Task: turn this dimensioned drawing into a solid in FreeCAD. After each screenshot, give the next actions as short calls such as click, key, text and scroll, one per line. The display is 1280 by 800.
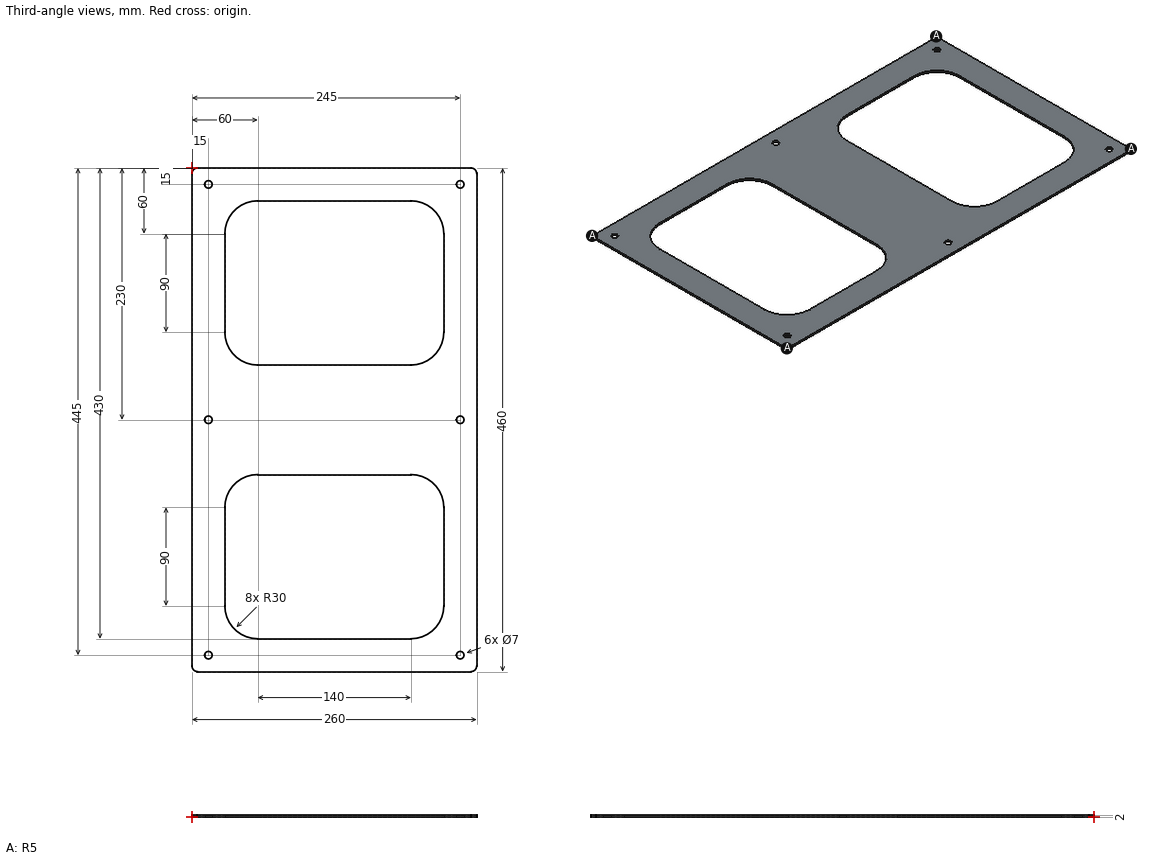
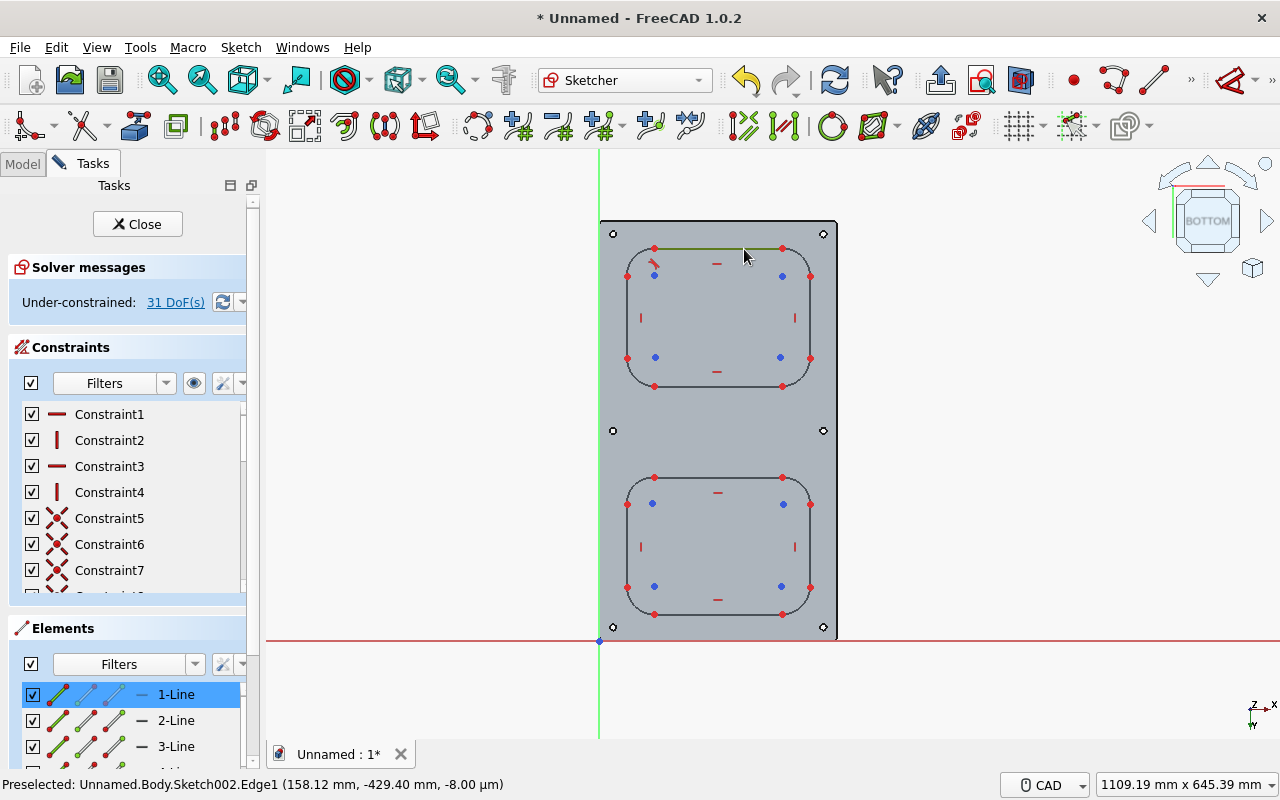
click(807, 264)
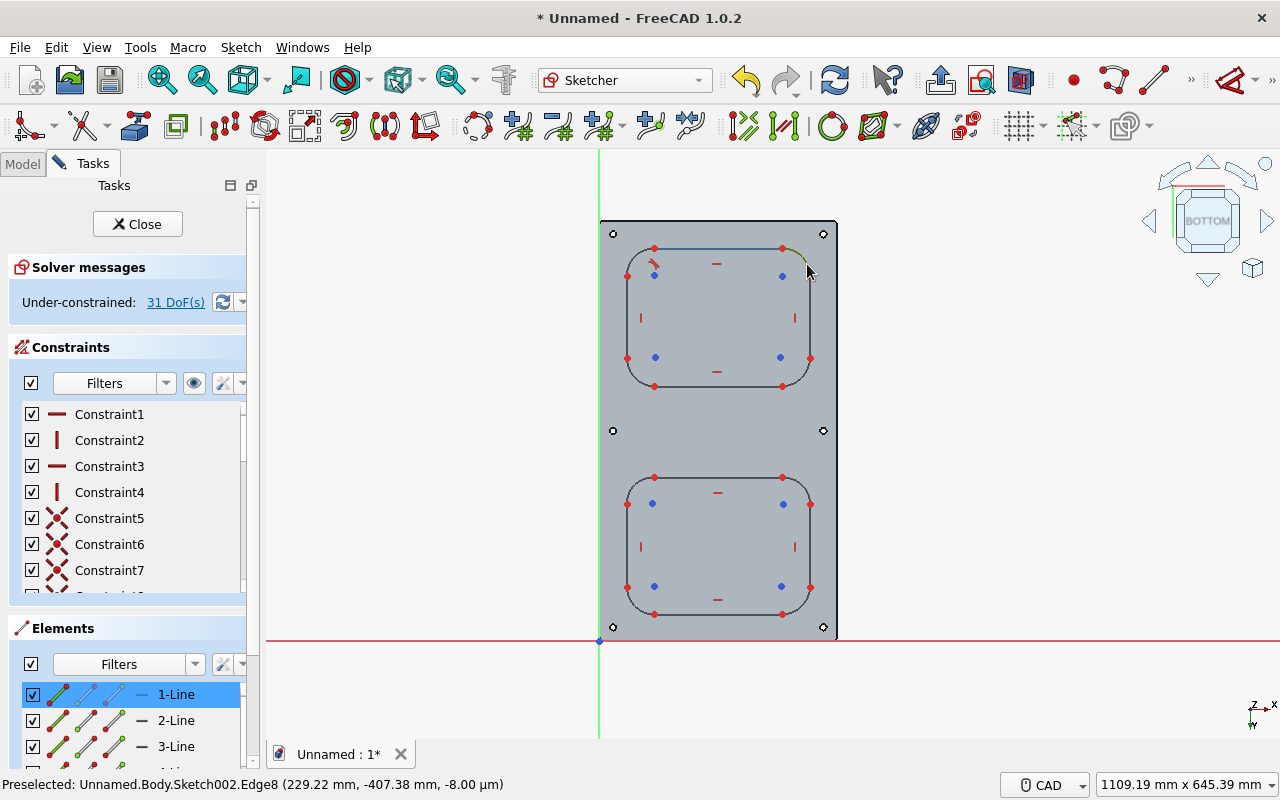
key(t)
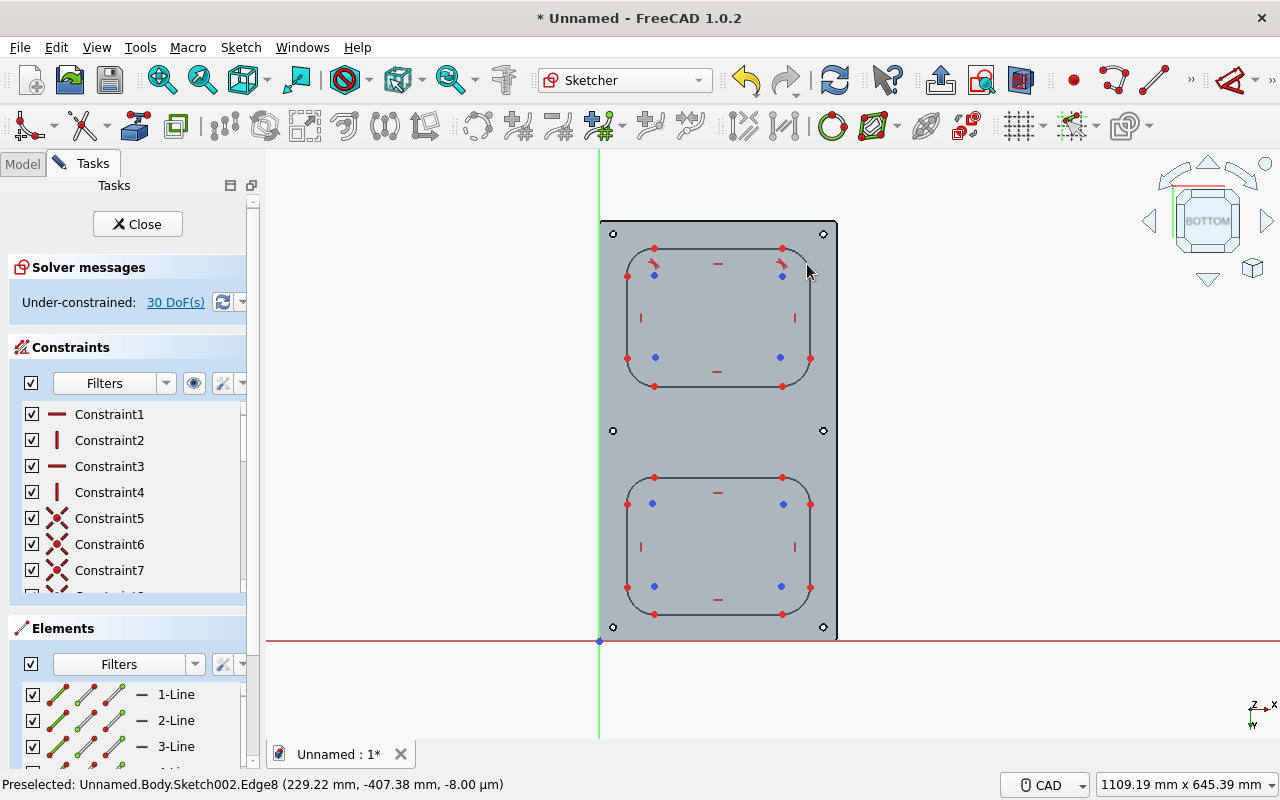
click(627, 301)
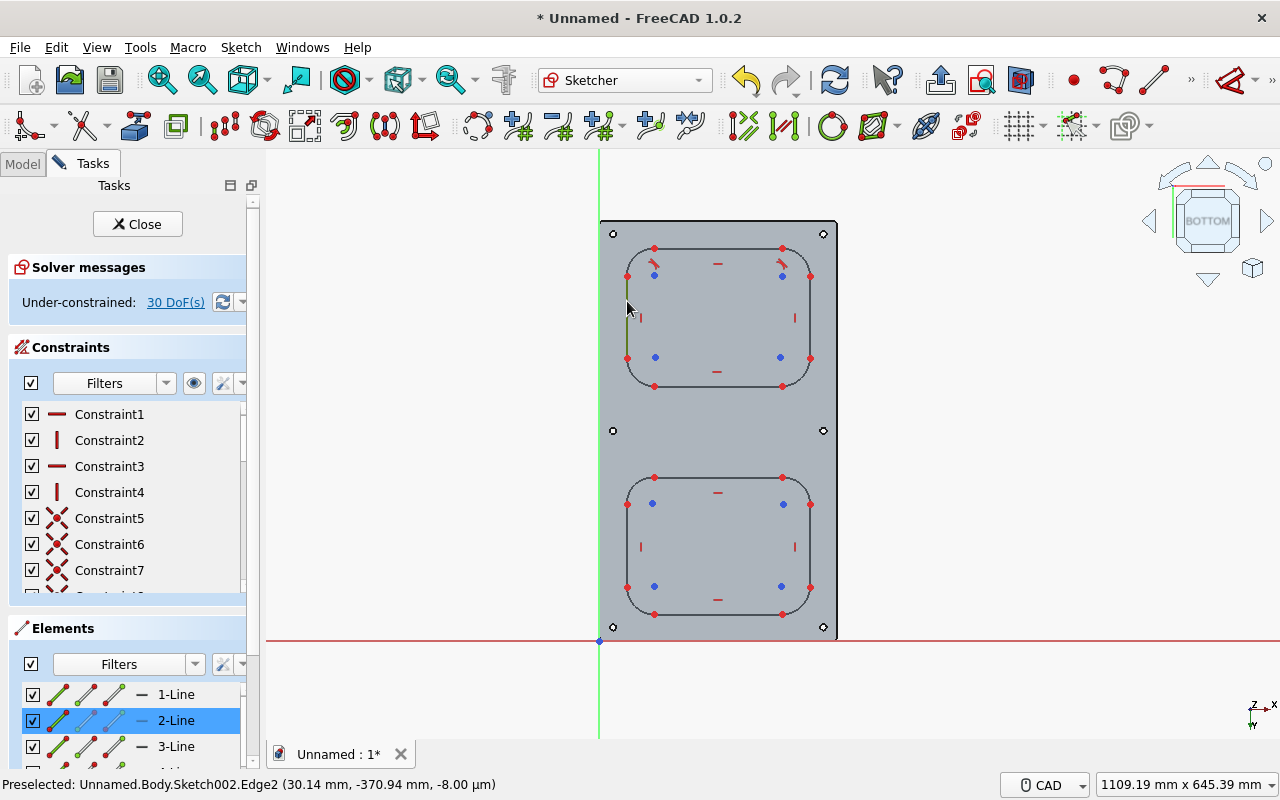
click(641, 252)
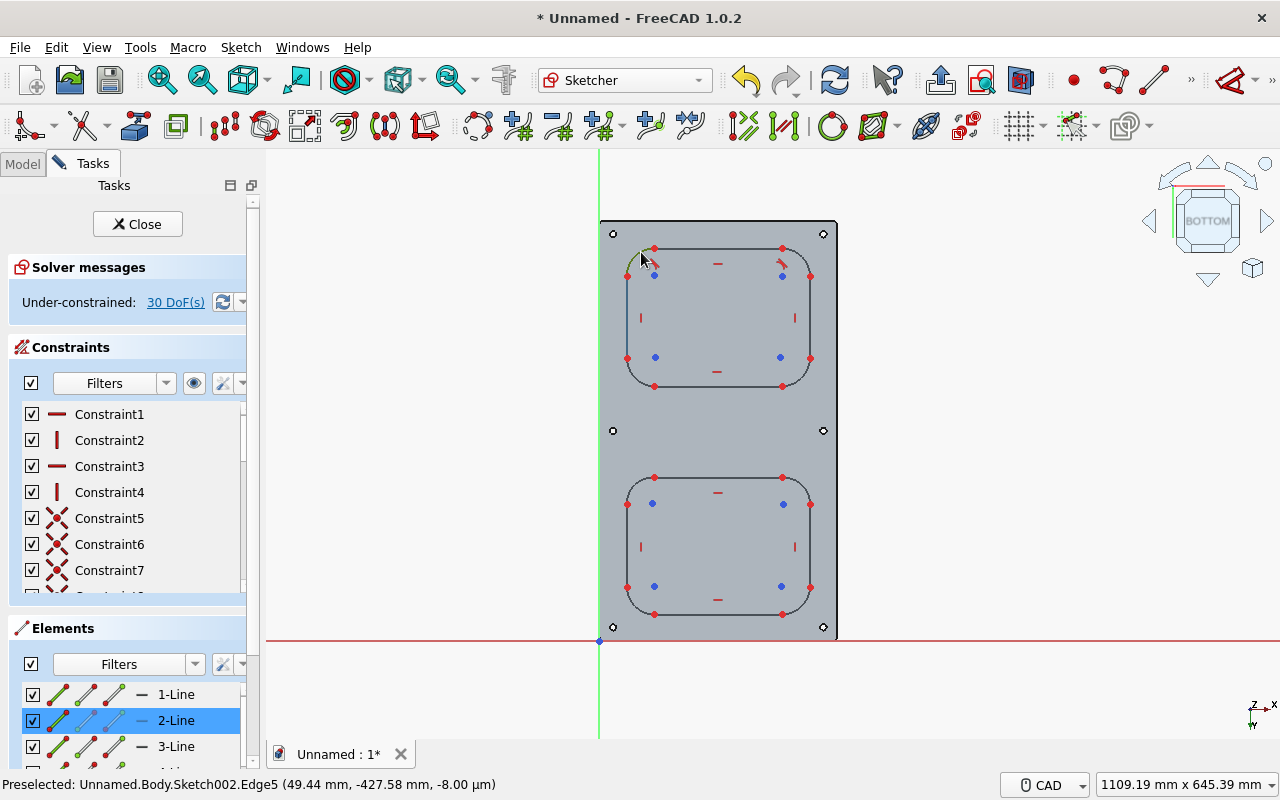
key(t)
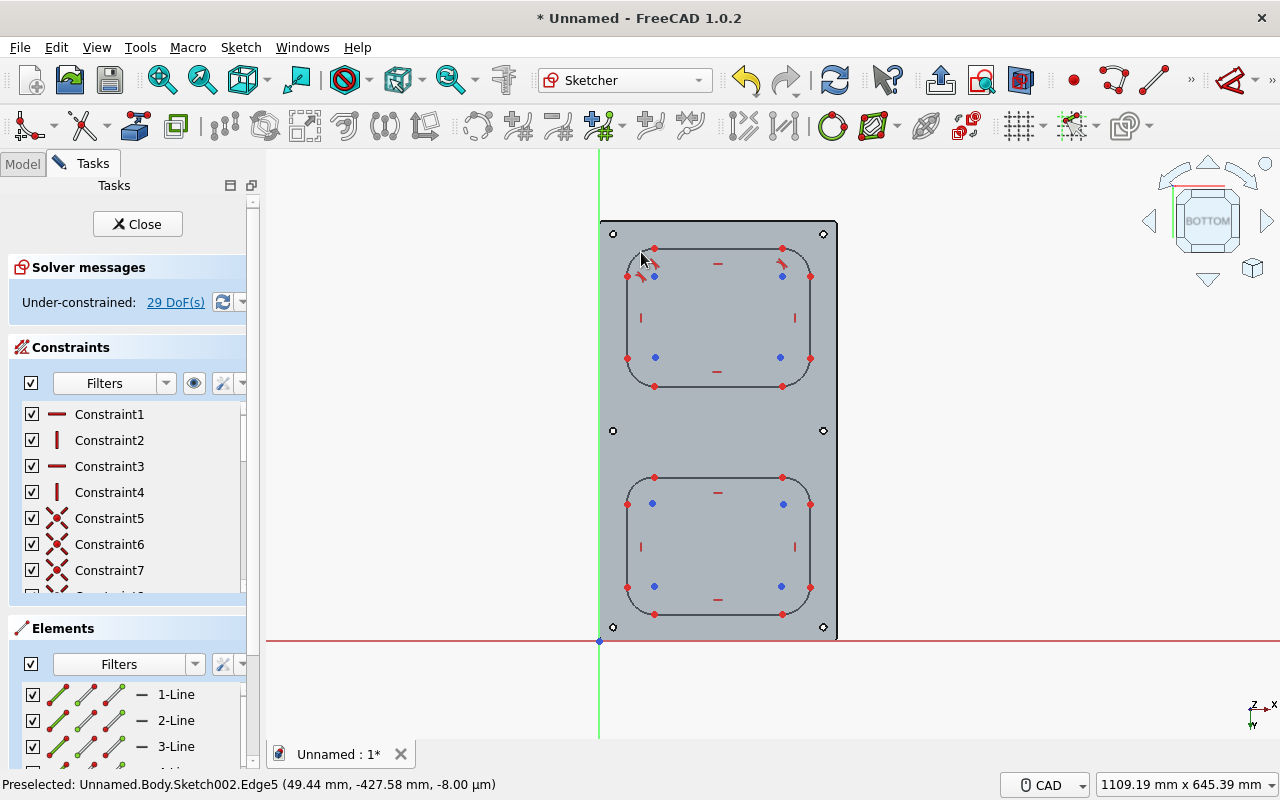
click(627, 301)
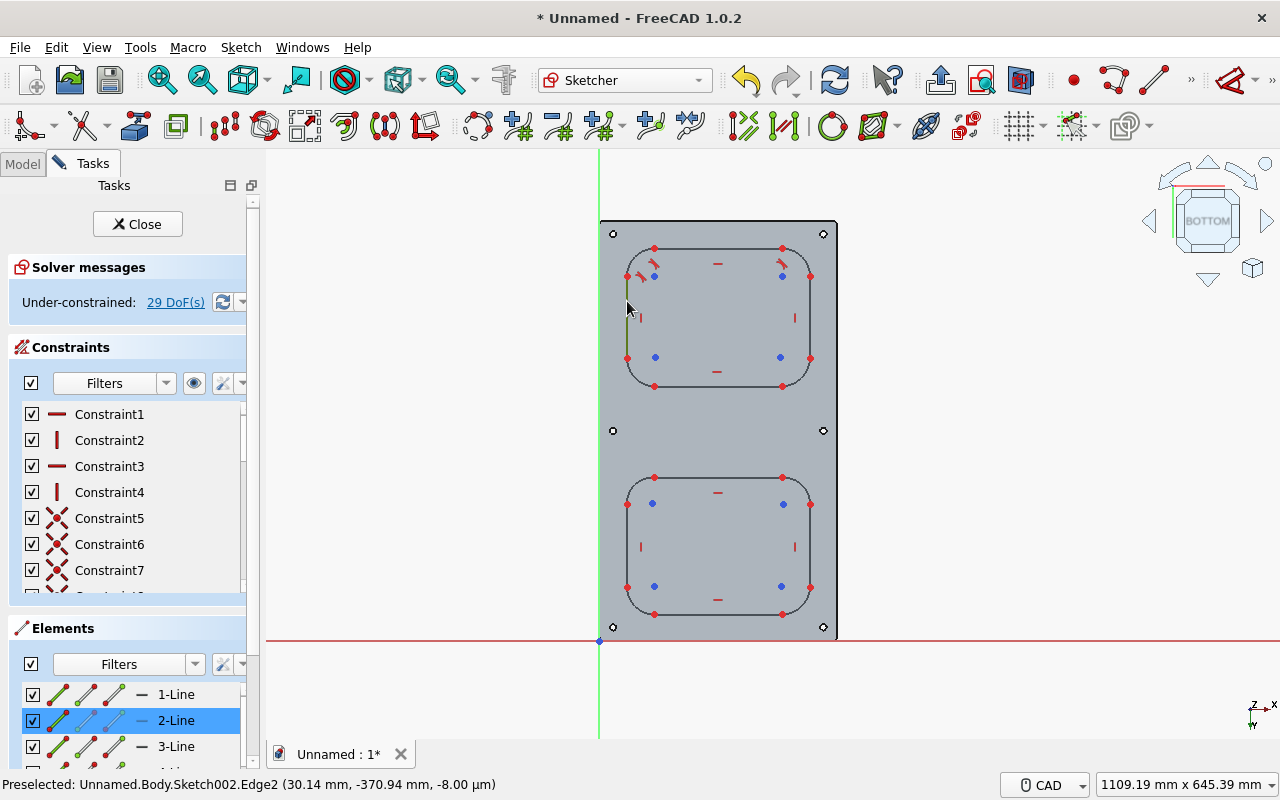
click(630, 371)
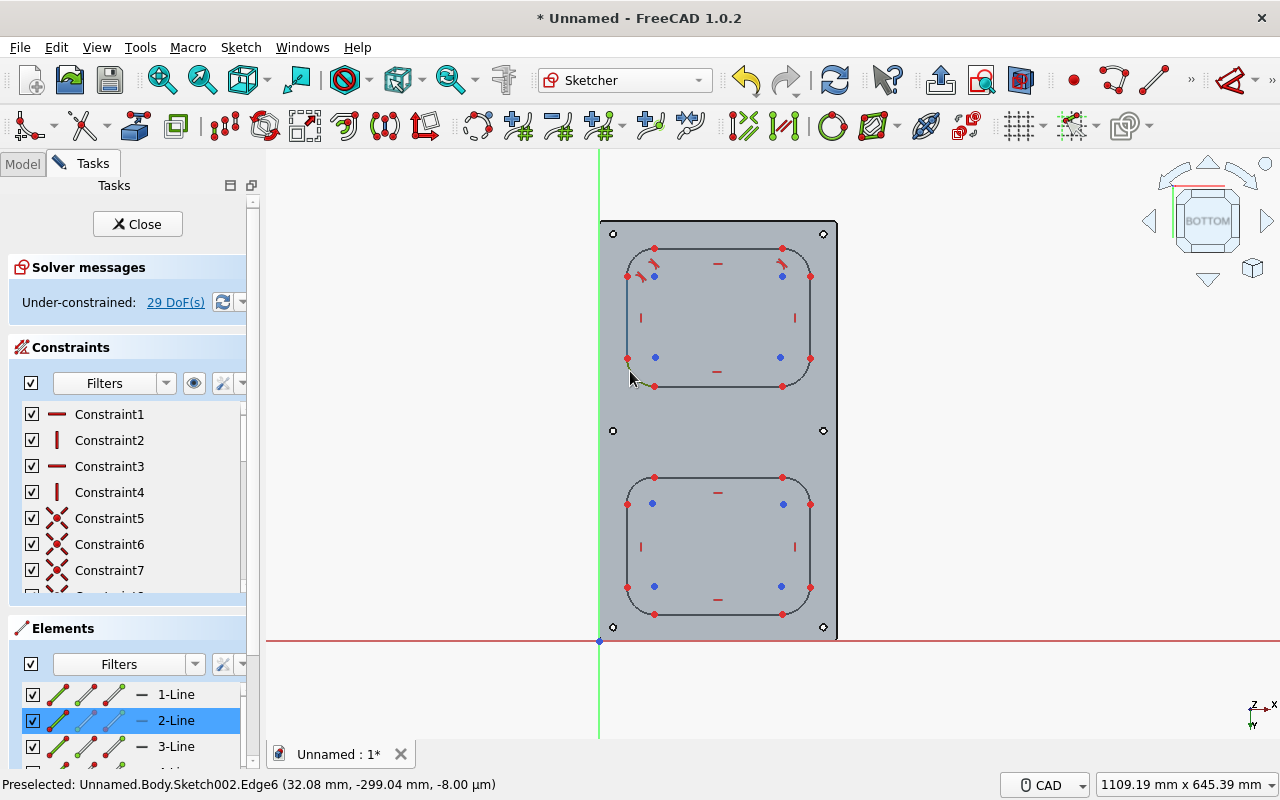
key(t)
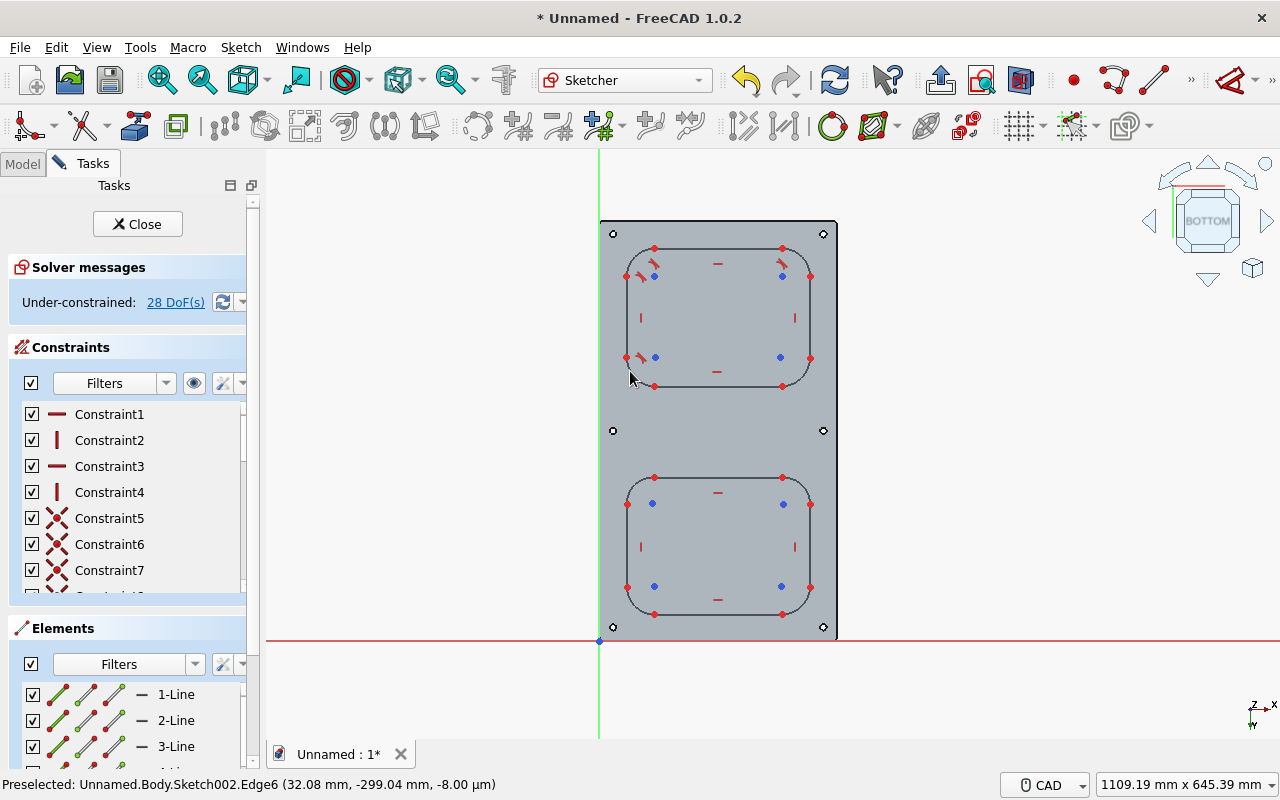
click(692, 387)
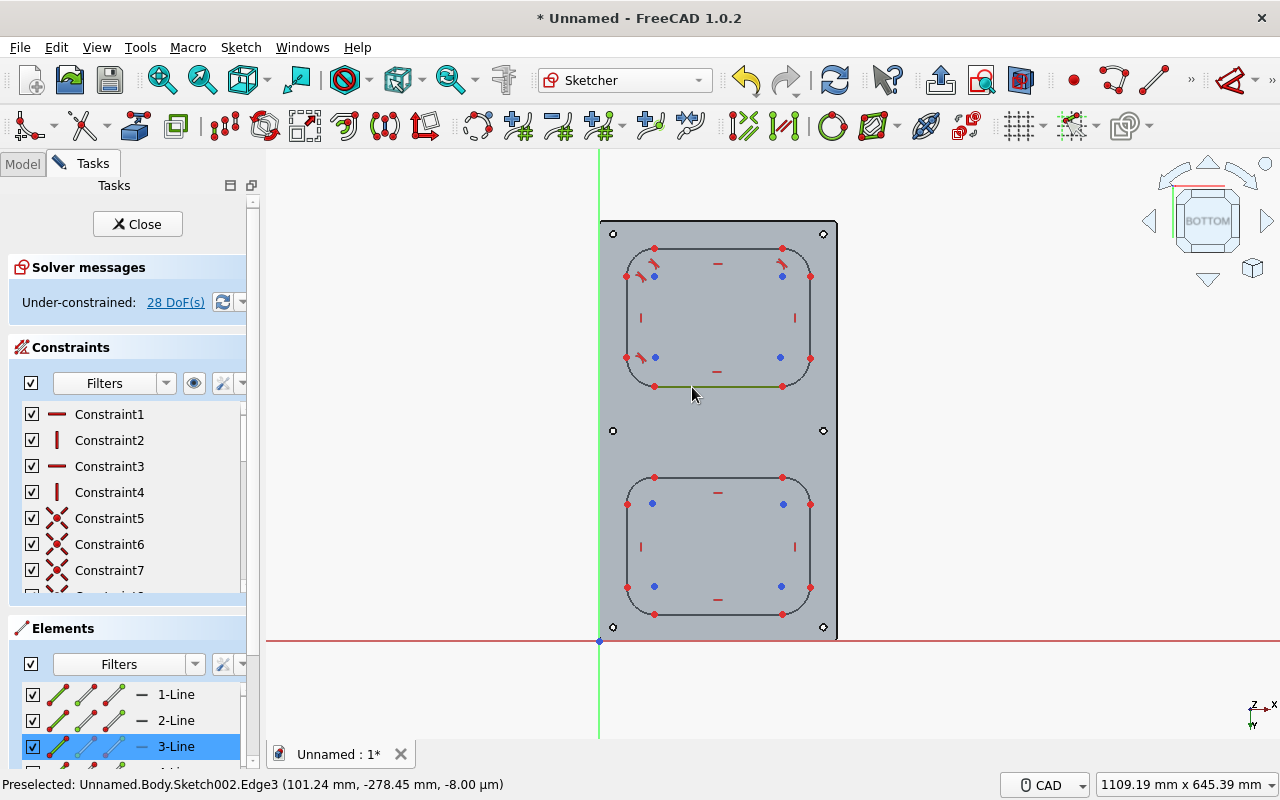
click(630, 370)